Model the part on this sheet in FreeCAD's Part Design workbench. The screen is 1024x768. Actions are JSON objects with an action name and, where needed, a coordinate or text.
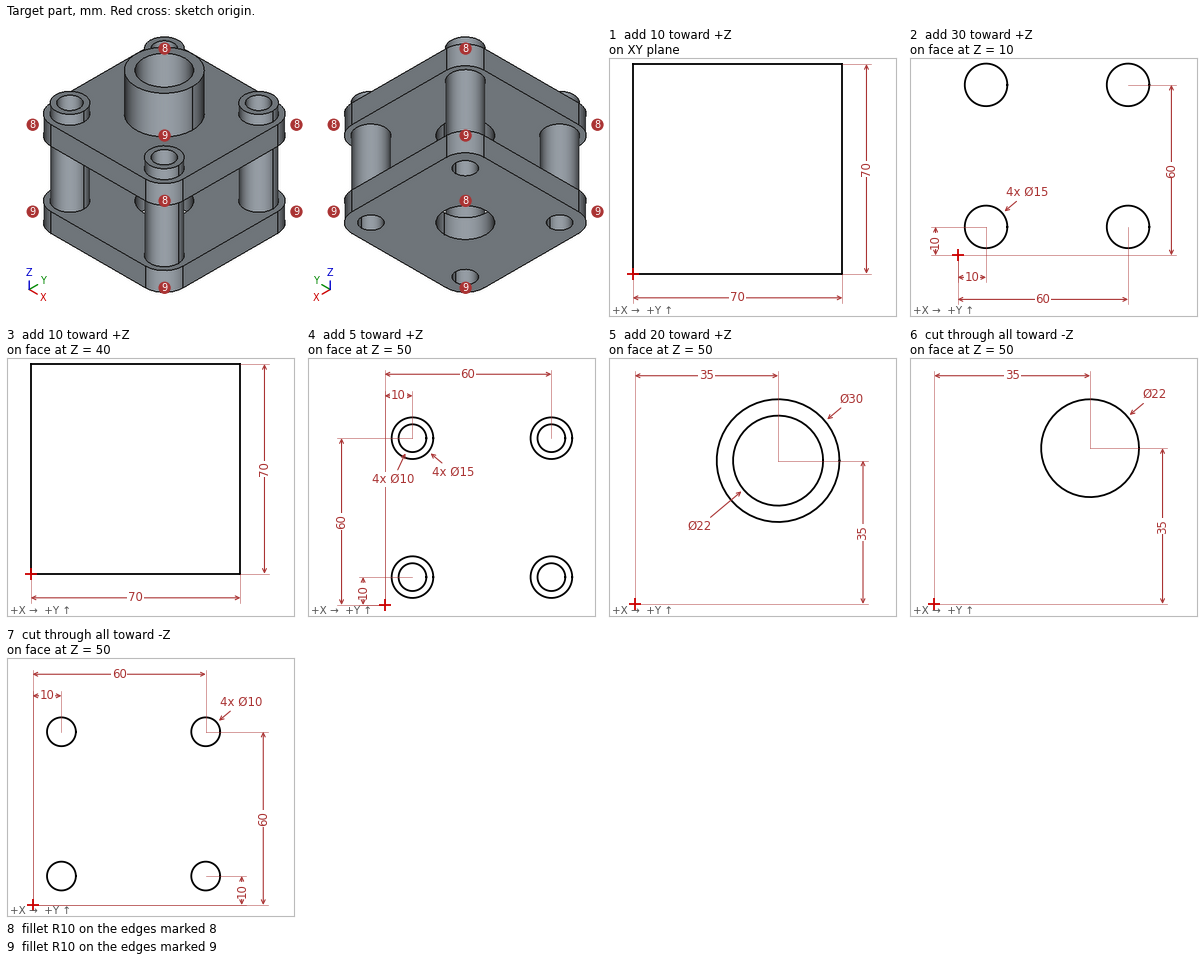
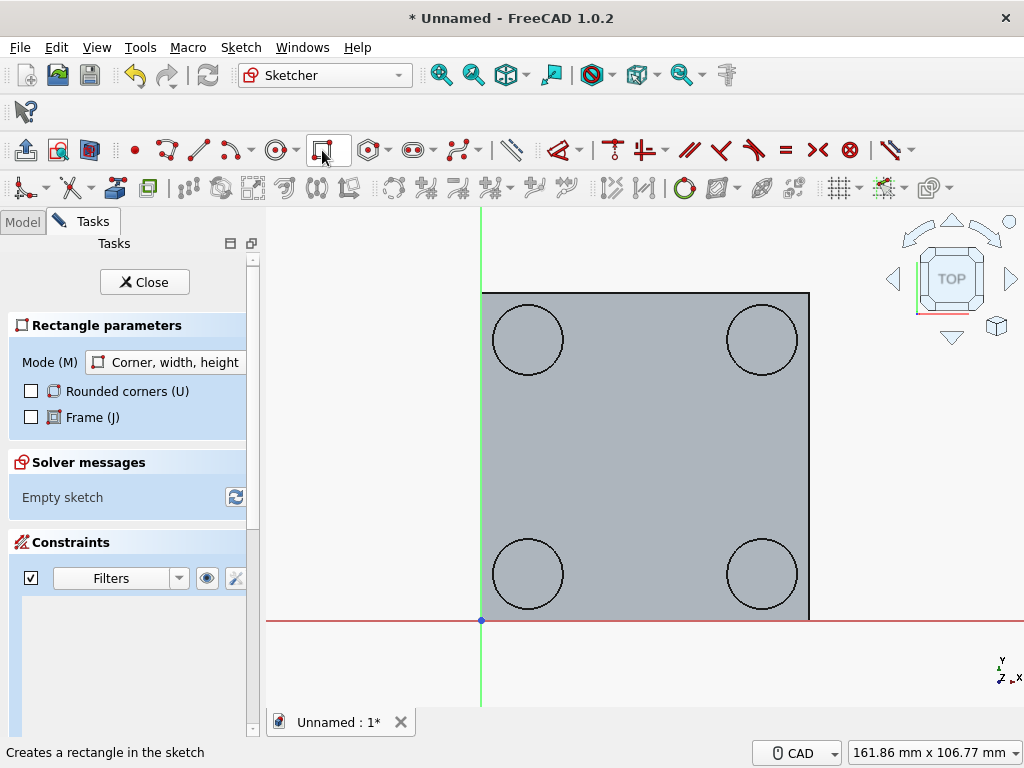
{"action": "left_click", "coordinate": [481, 621]}
{"action": "left_click", "coordinate": [809, 293]}
{"action": "key", "text": "Escape"}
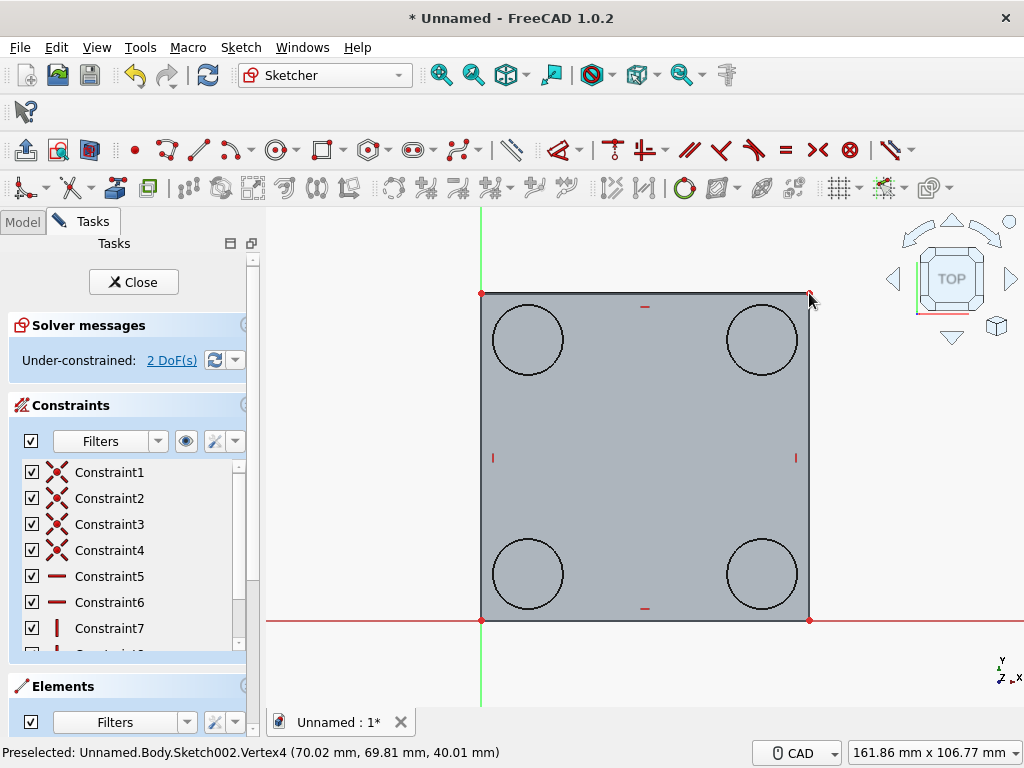
{"action": "key", "text": "d"}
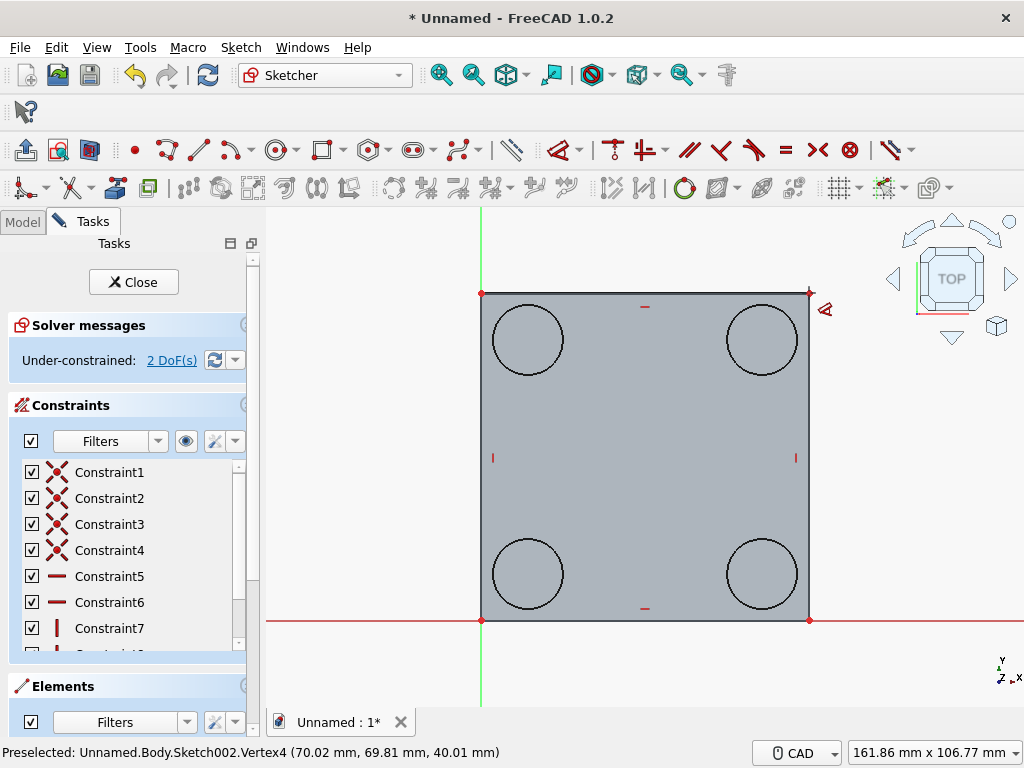
{"action": "left_click", "coordinate": [579, 621]}
{"action": "left_click", "coordinate": [645, 655]}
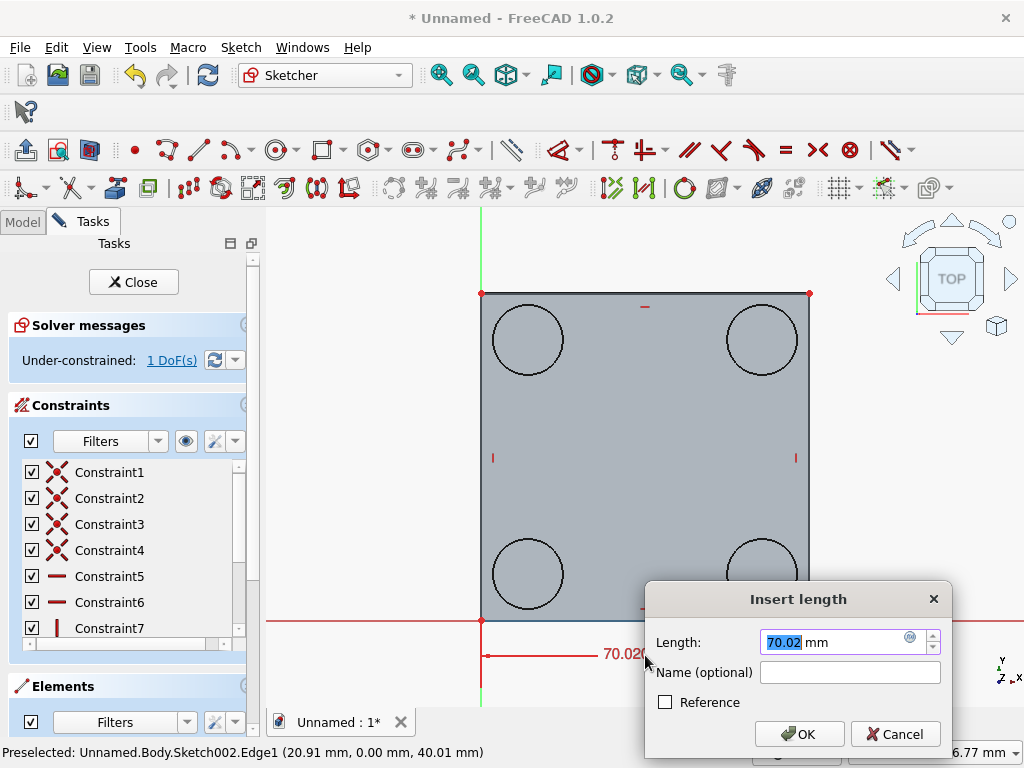
{"action": "type", "text": "70"}
{"action": "key", "text": "Return"}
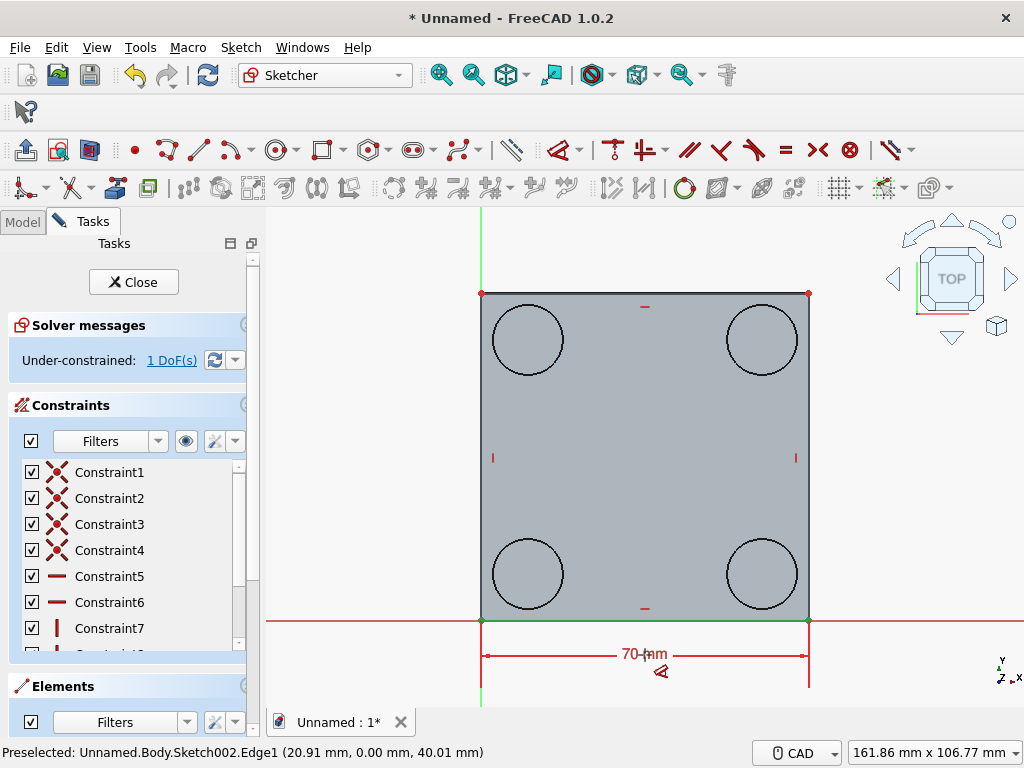
{"action": "left_click", "coordinate": [809, 523]}
{"action": "left_click", "coordinate": [843, 457]}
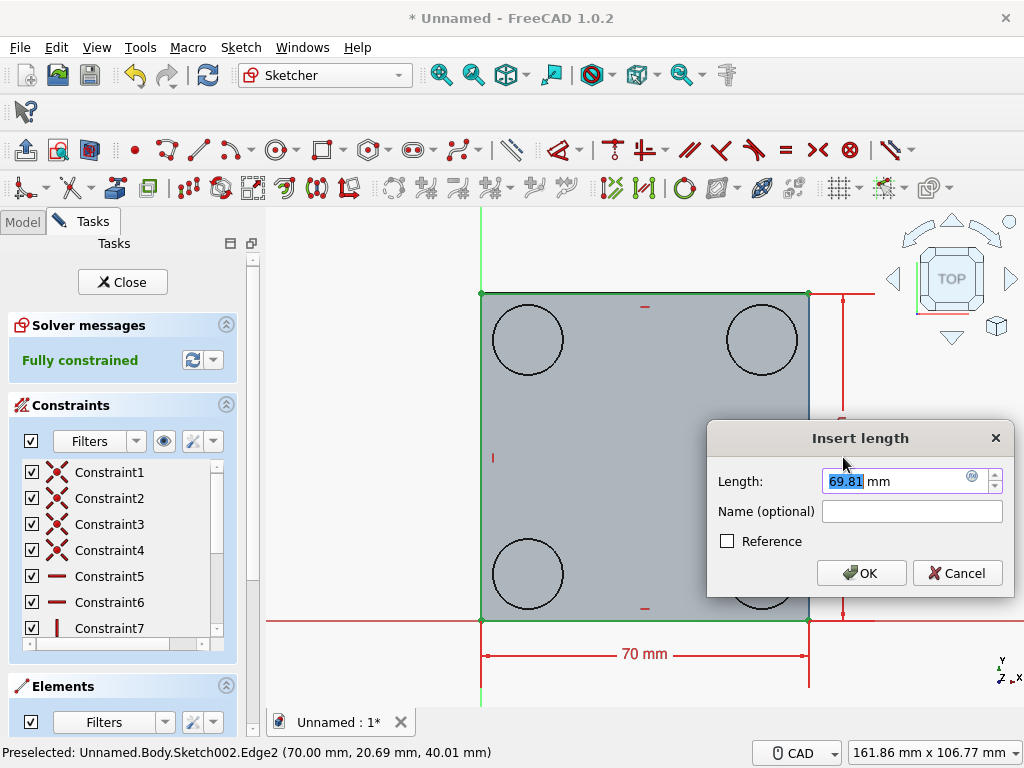
{"action": "type", "text": "70"}
{"action": "key", "text": "Return"}
{"action": "key", "text": "Escape"}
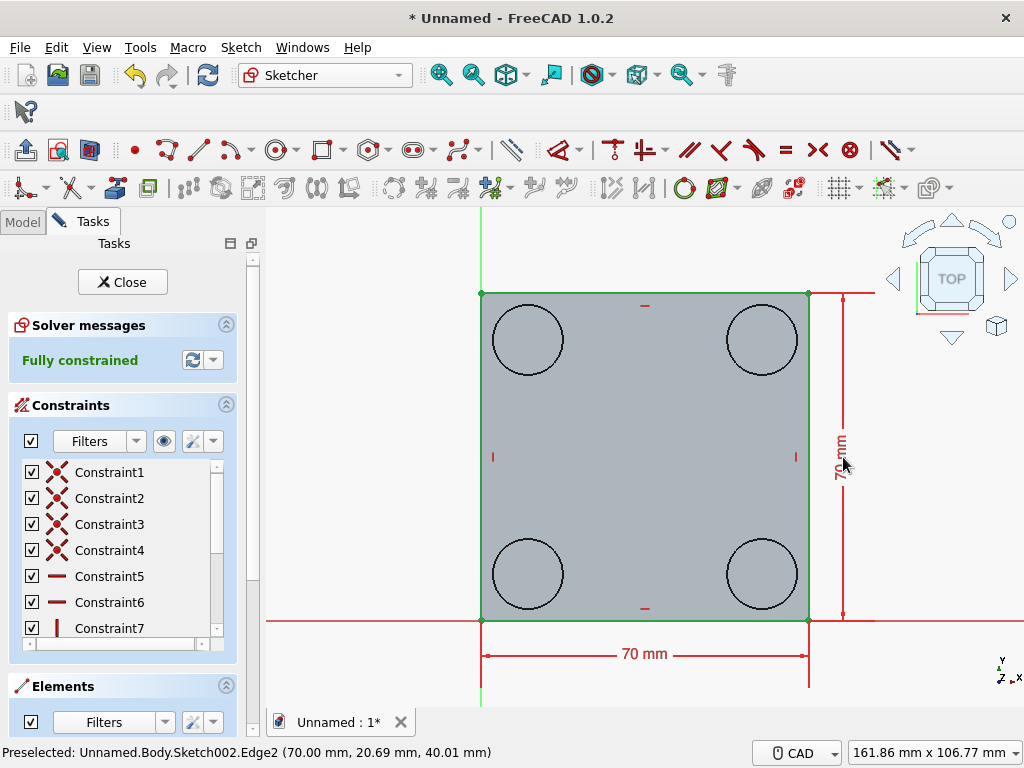
{"action": "left_click", "coordinate": [123, 282]}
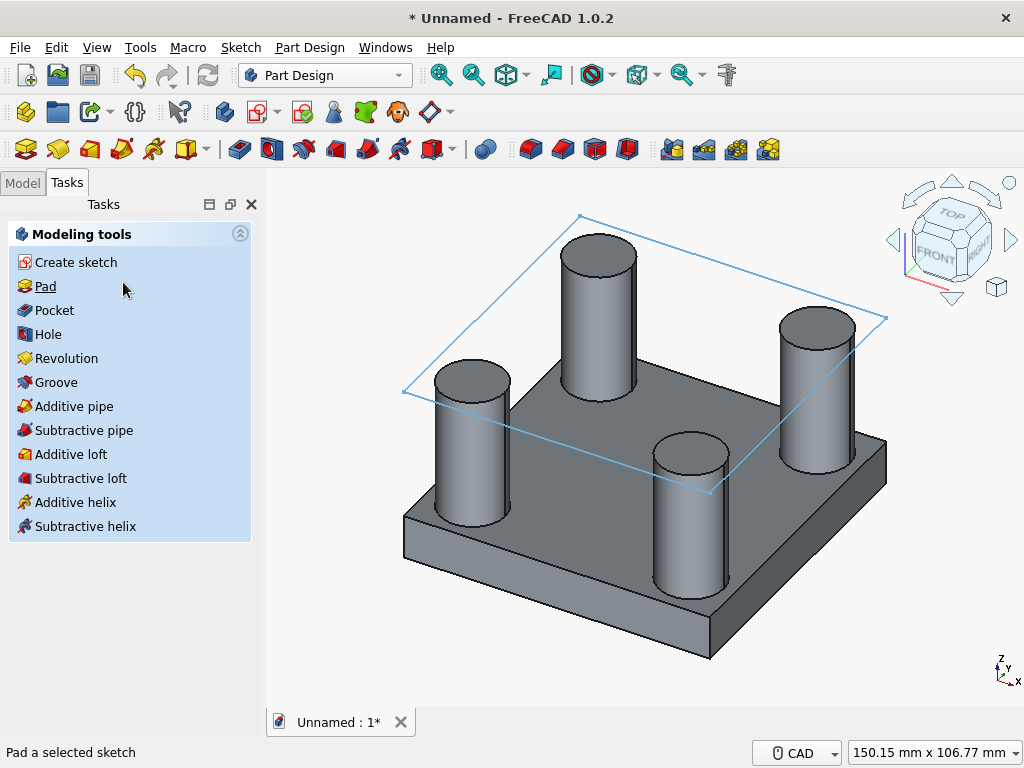
{"action": "left_click", "coordinate": [26, 150]}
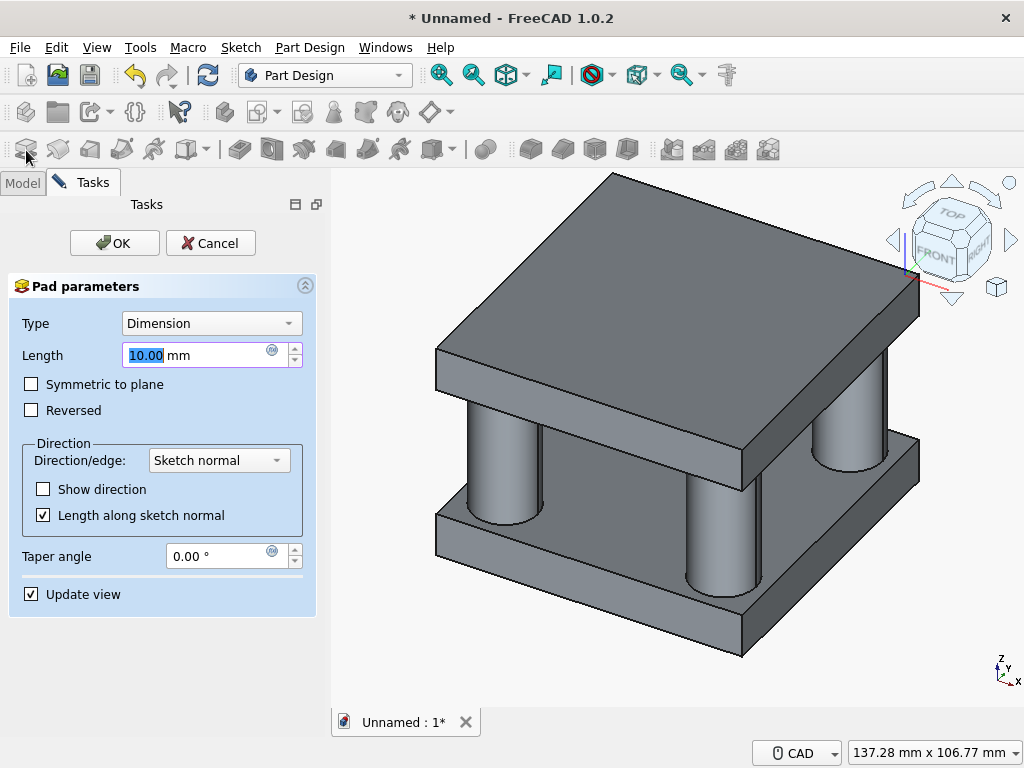
{"action": "type", "text": "10"}
{"action": "key", "text": "Tab"}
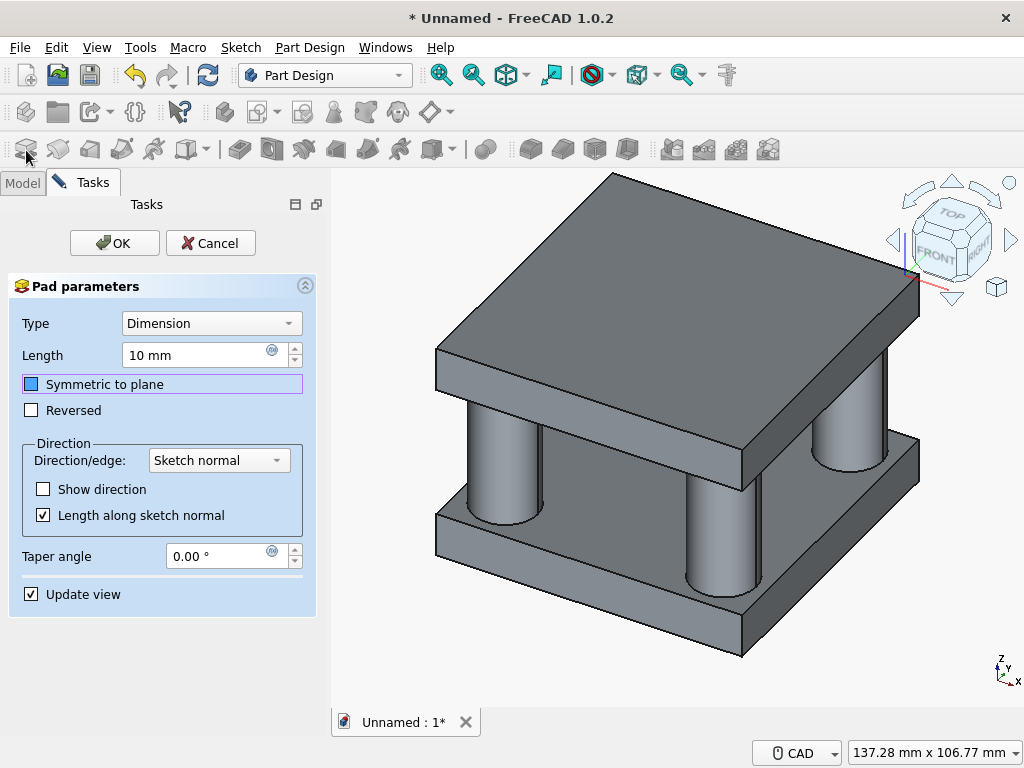
{"action": "left_click", "coordinate": [115, 243]}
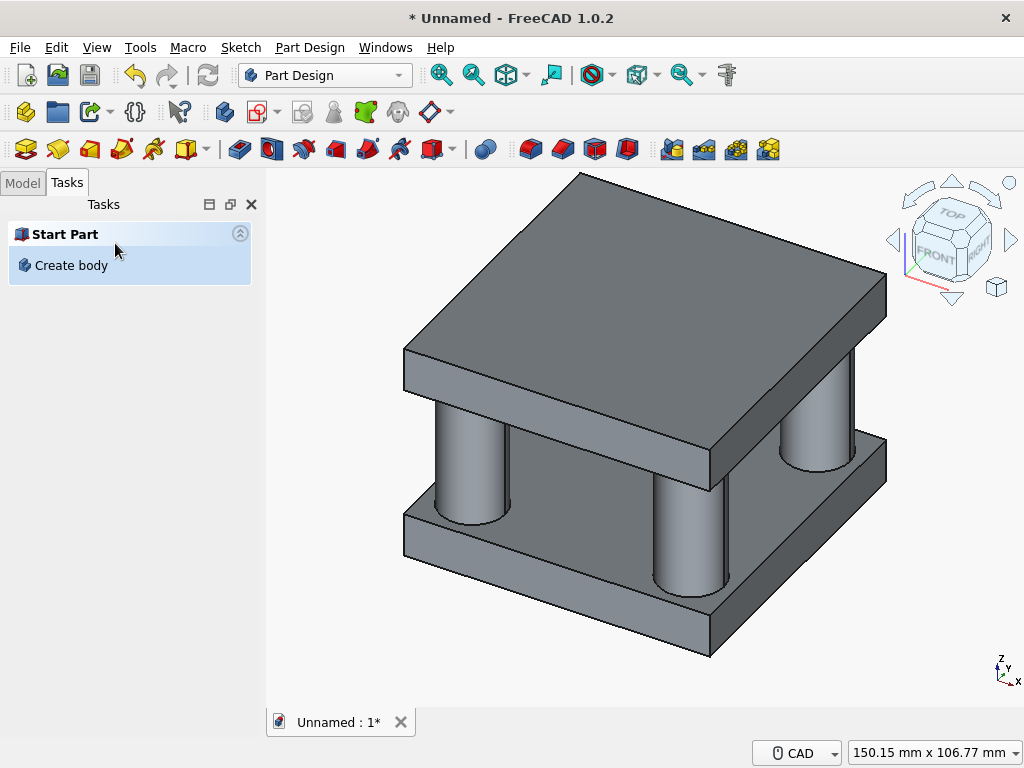
{"action": "left_click", "coordinate": [645, 310]}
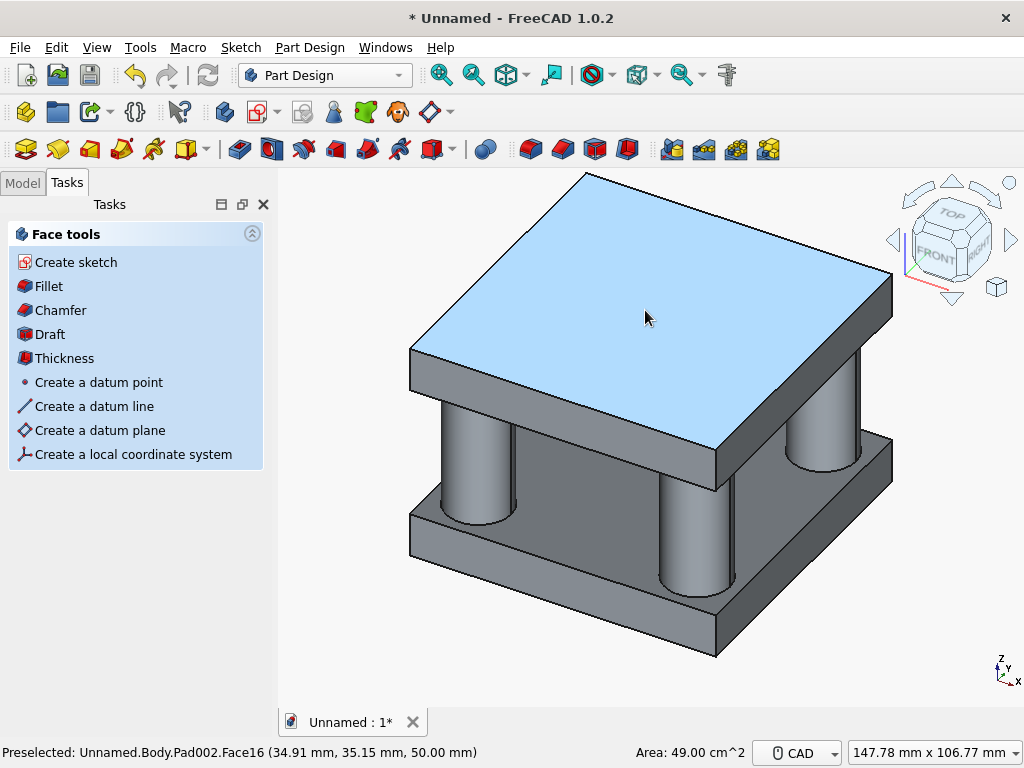
{"action": "left_click", "coordinate": [258, 112]}